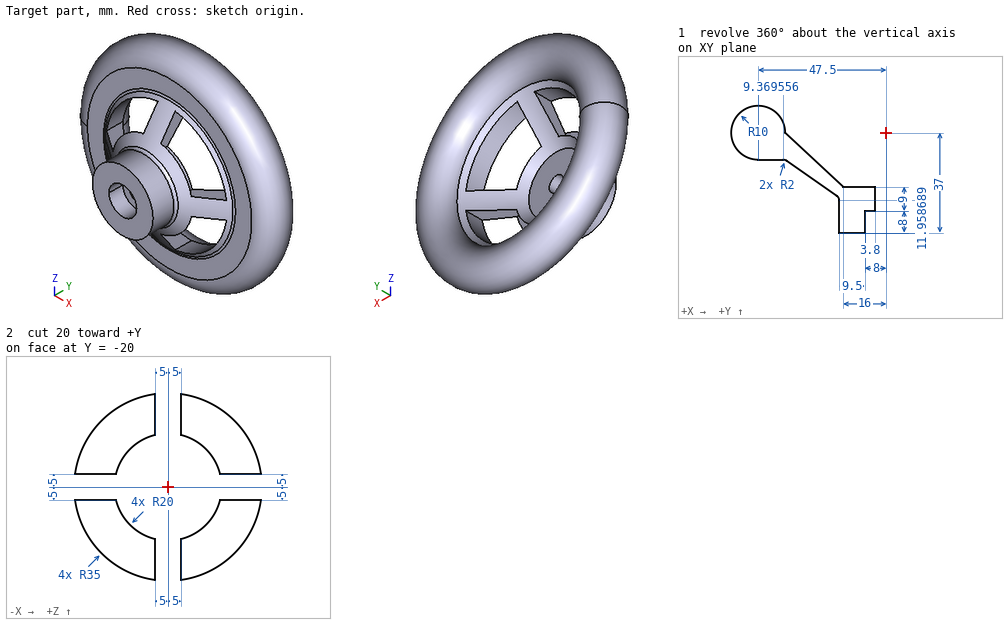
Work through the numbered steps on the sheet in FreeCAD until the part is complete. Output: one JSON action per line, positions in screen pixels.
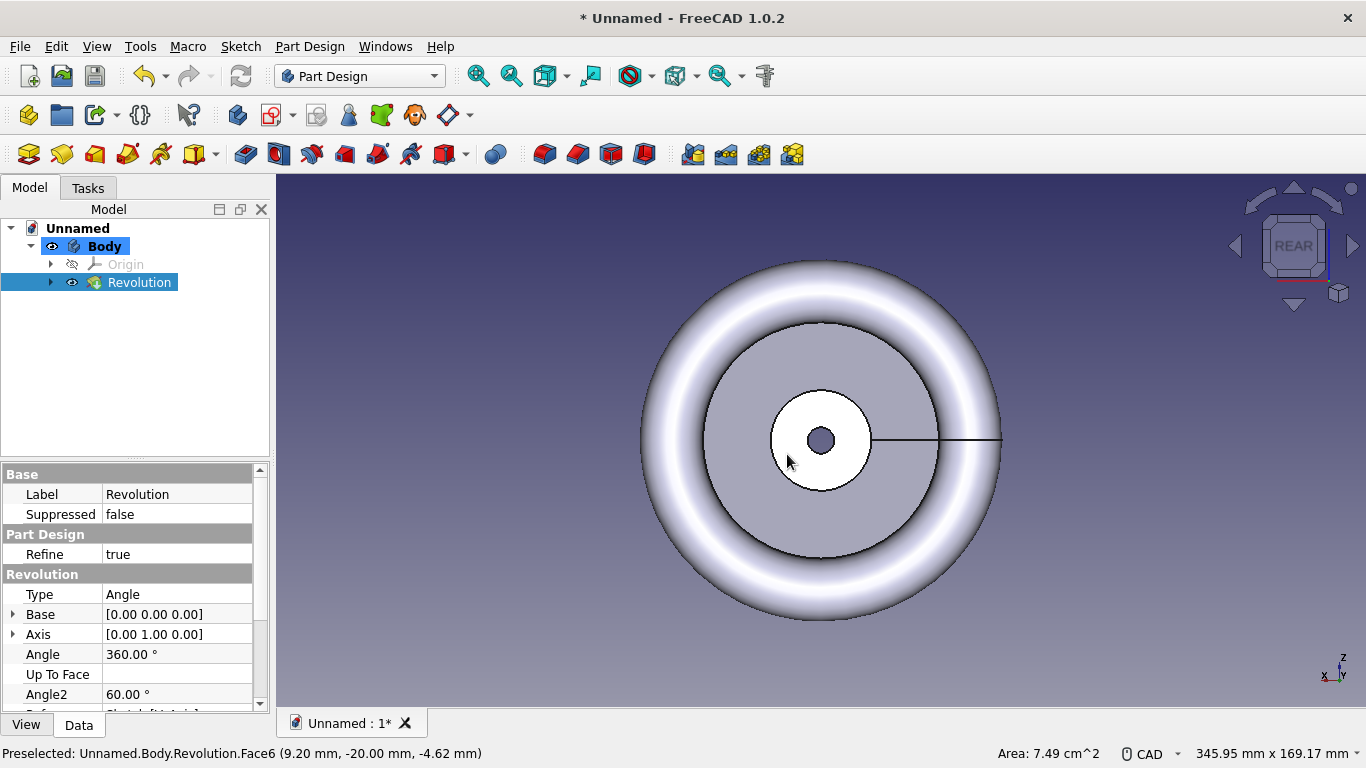
{"action": "left_click", "coordinate": [270, 116]}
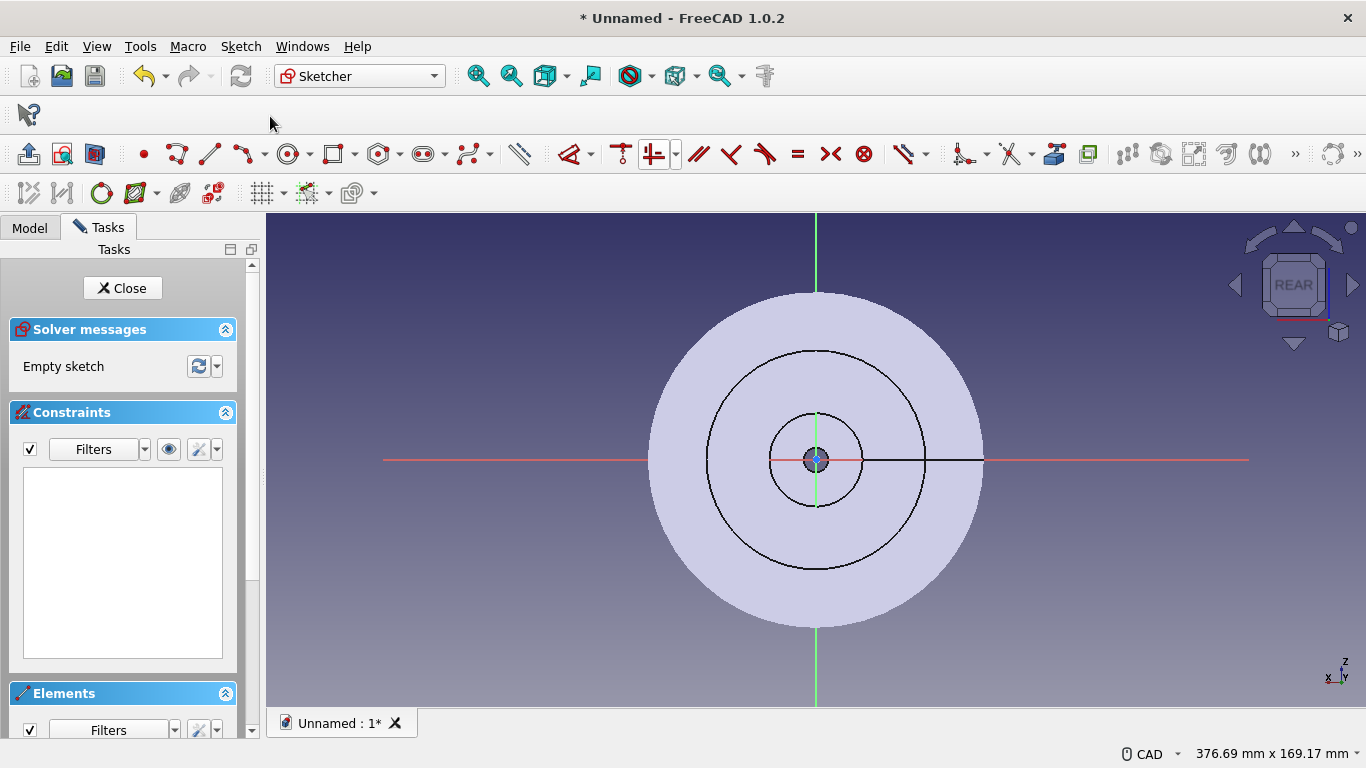
{"action": "scroll", "coordinate": [955, 460], "scroll_direction": "up", "scroll_amount": 2}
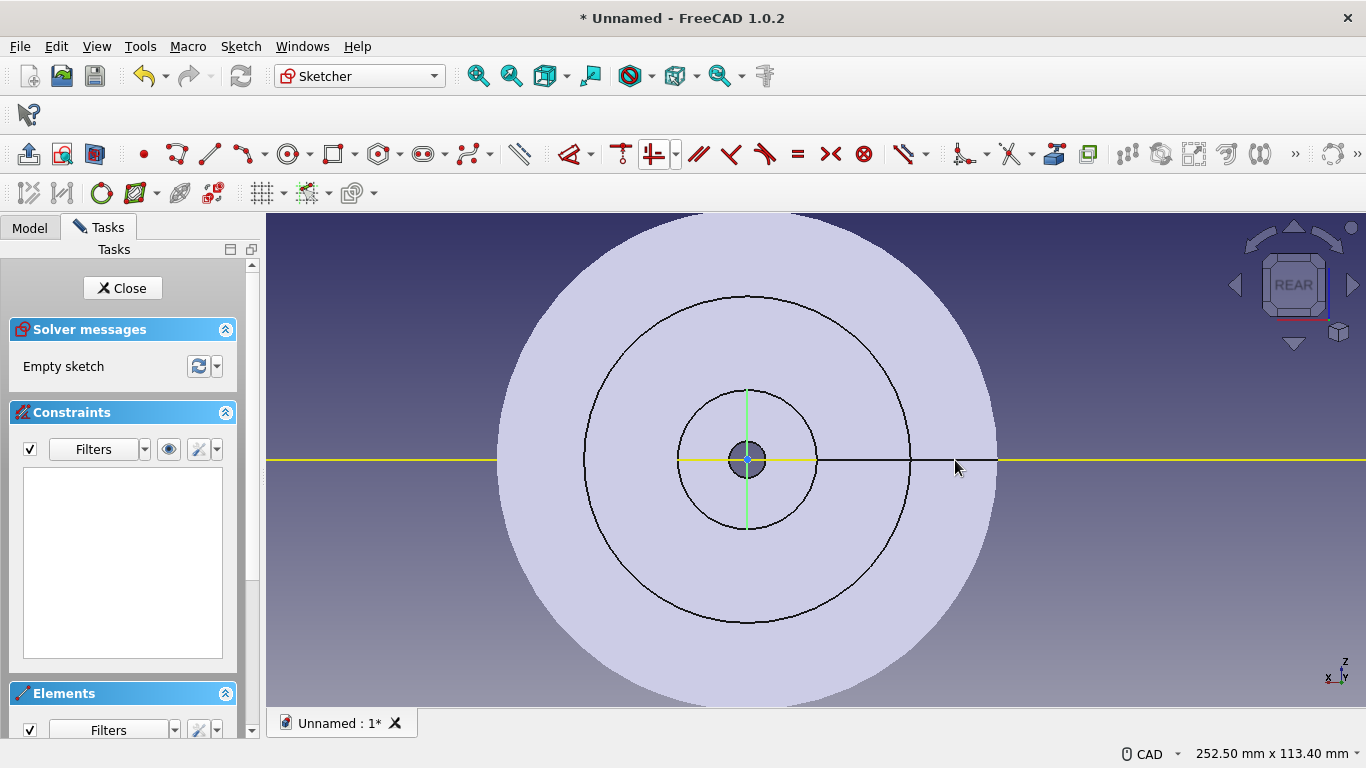
{"action": "left_click", "coordinate": [210, 154]}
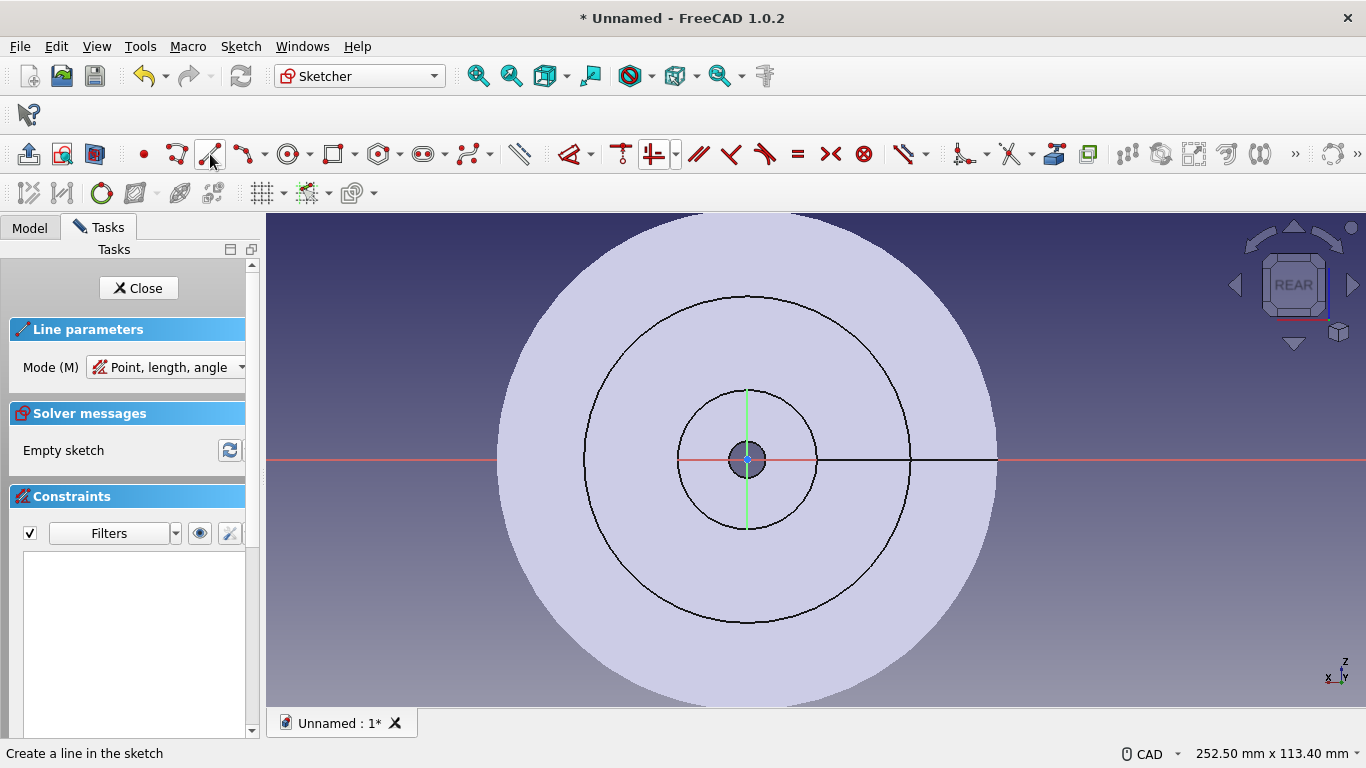
{"action": "left_click", "coordinate": [663, 481]}
{"action": "left_click", "coordinate": [596, 481]}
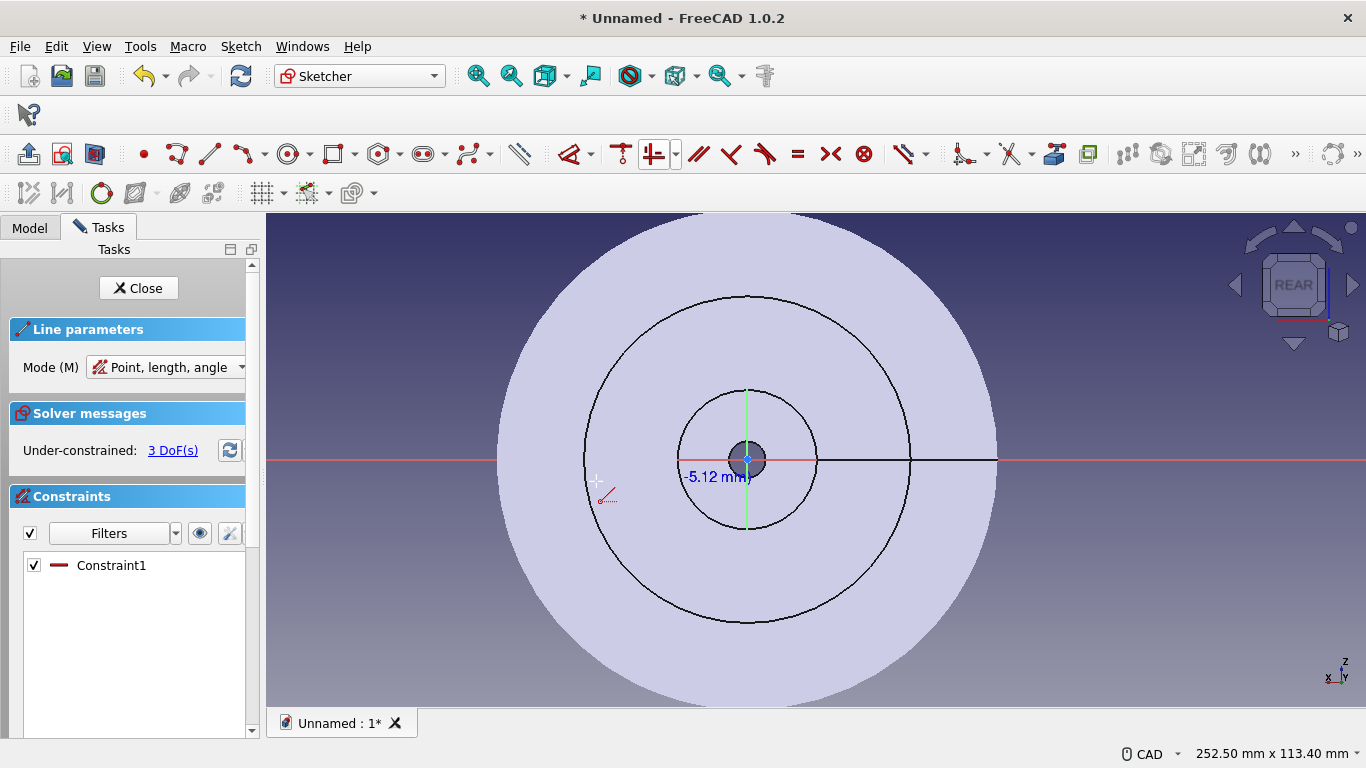
{"action": "left_click", "coordinate": [726, 611]}
{"action": "left_click", "coordinate": [726, 544]}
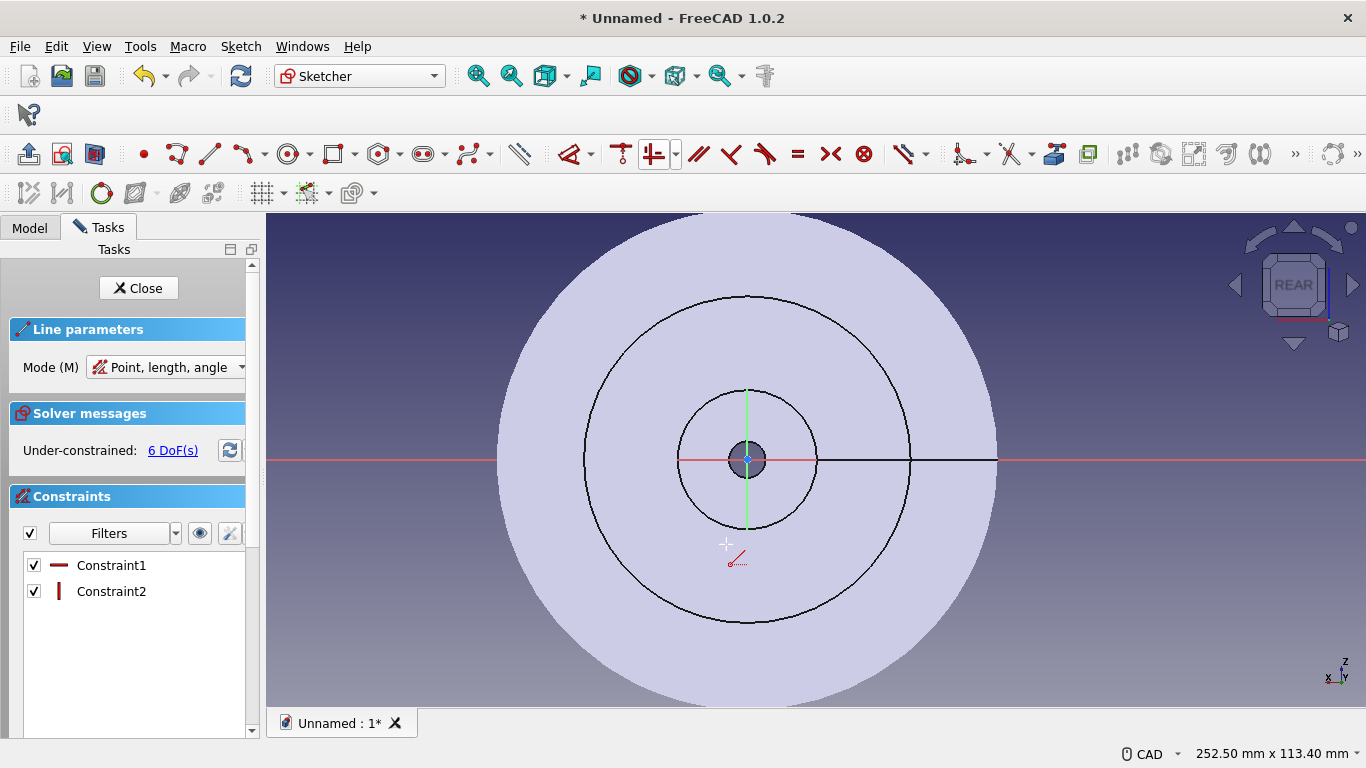
{"action": "key", "text": "g 3 a"}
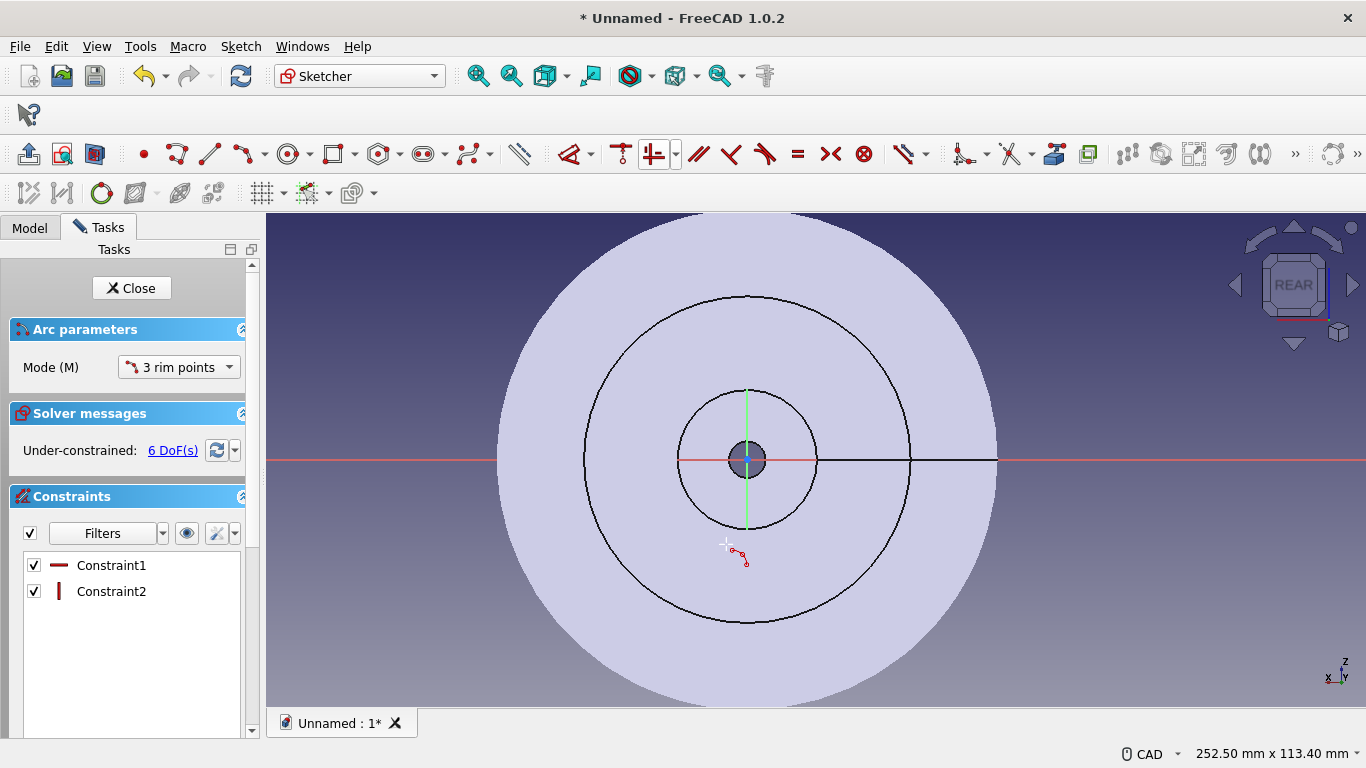
{"action": "left_click", "coordinate": [596, 482]}
{"action": "left_click", "coordinate": [726, 612]}
{"action": "left_click", "coordinate": [640, 568]}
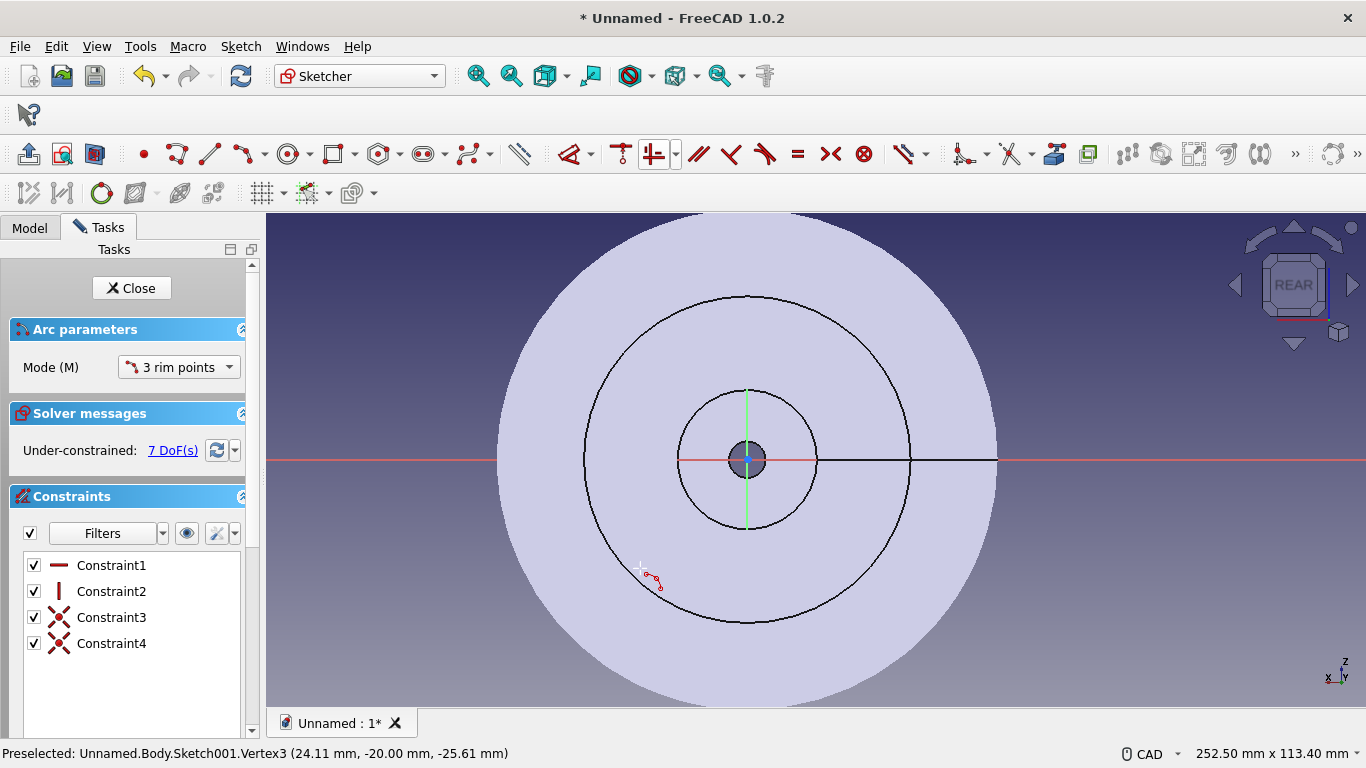
{"action": "left_click", "coordinate": [726, 545]}
{"action": "left_click", "coordinate": [663, 482]}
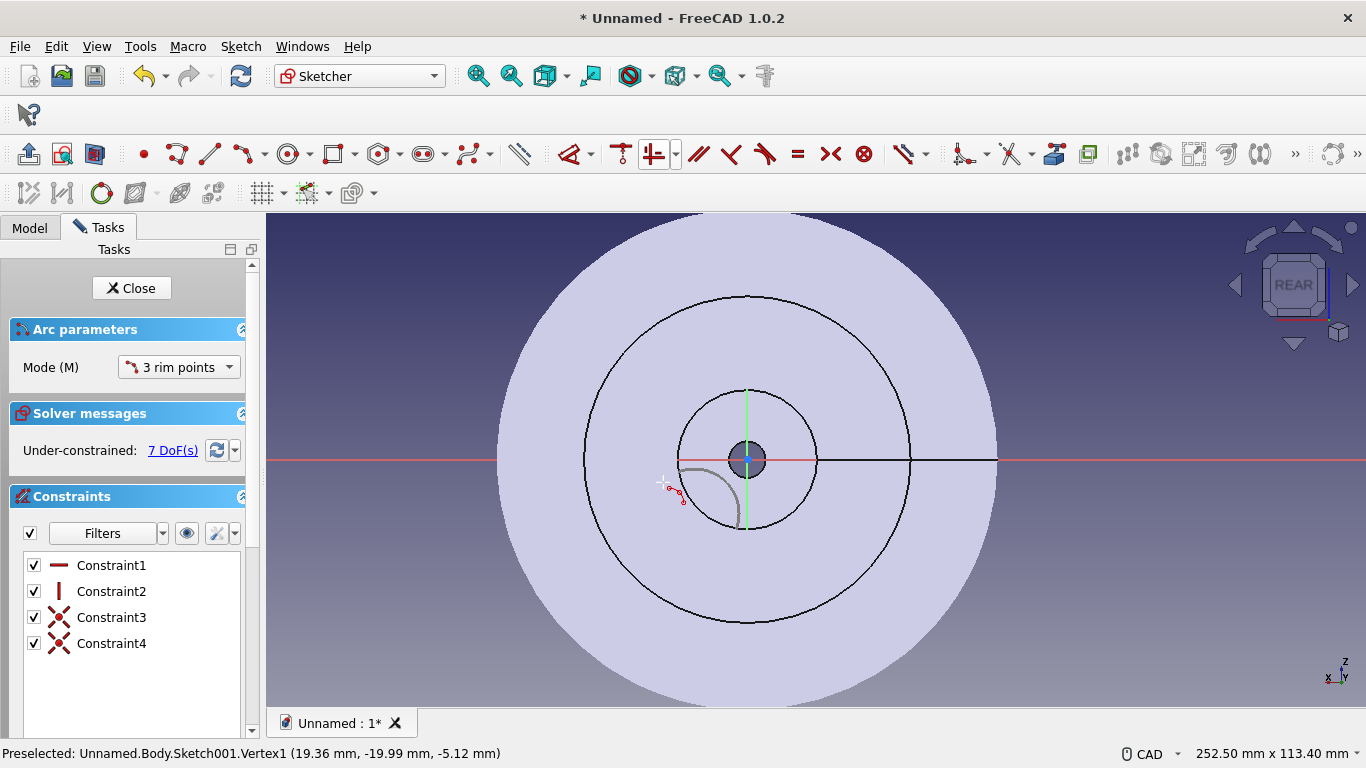
{"action": "scroll", "coordinate": [686, 521], "scroll_direction": "up", "scroll_amount": 2}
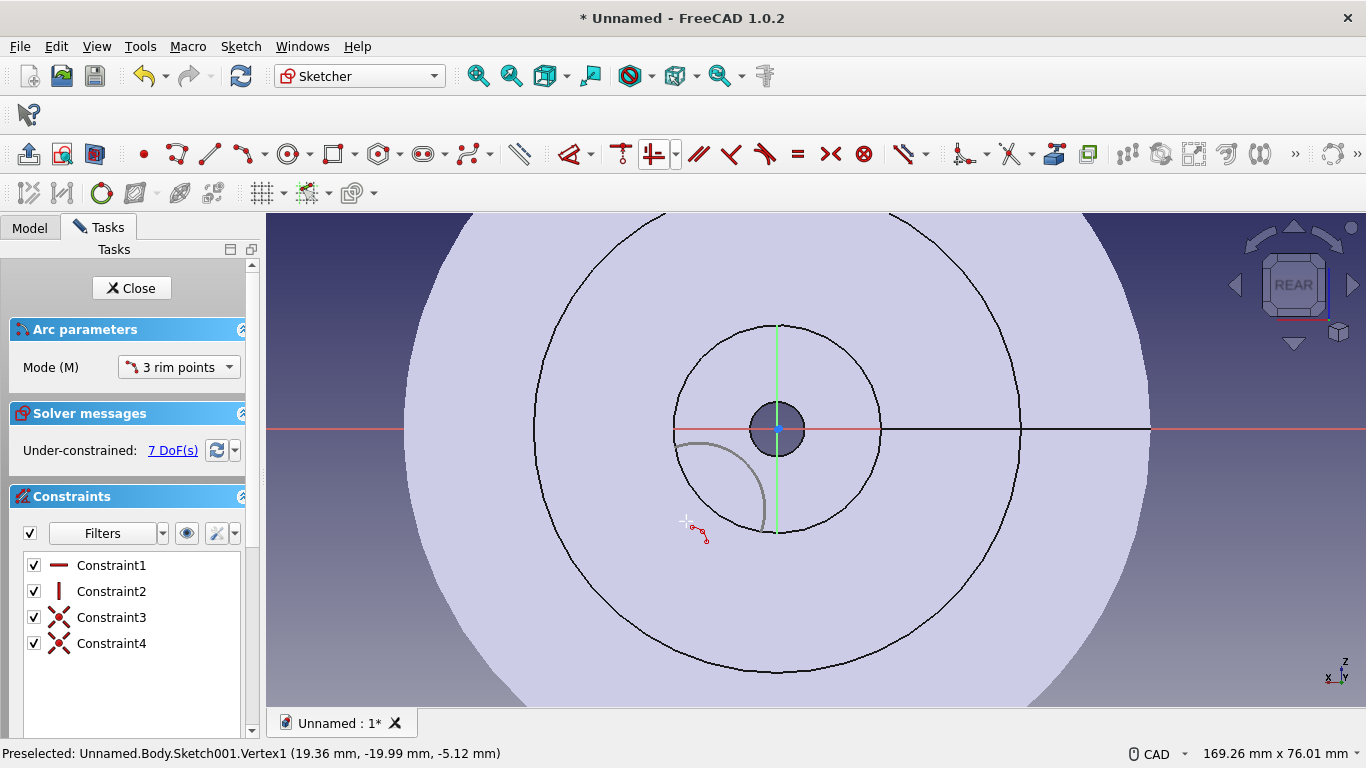
{"action": "left_click", "coordinate": [685, 521]}